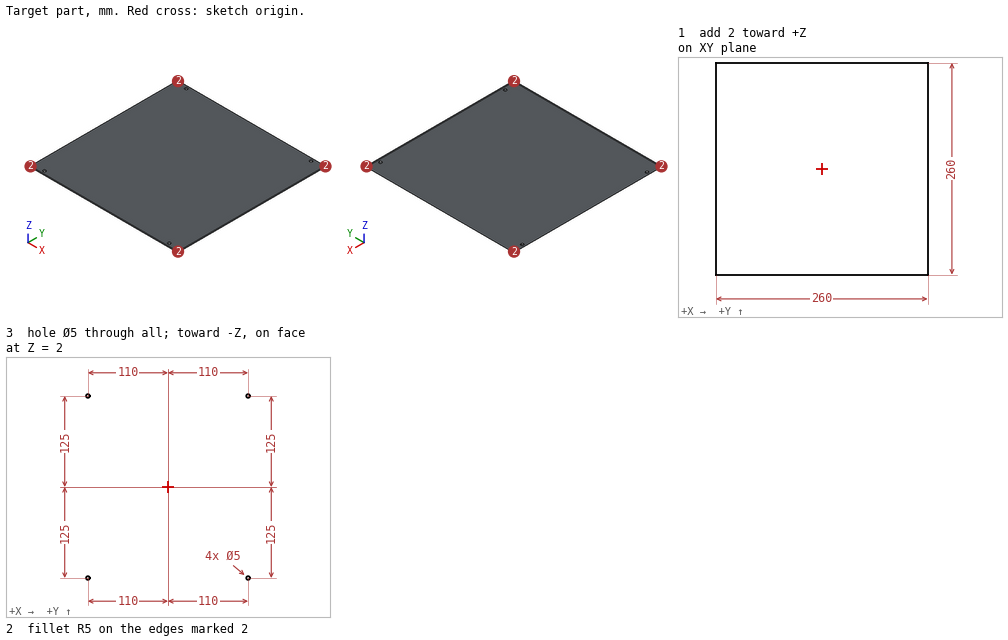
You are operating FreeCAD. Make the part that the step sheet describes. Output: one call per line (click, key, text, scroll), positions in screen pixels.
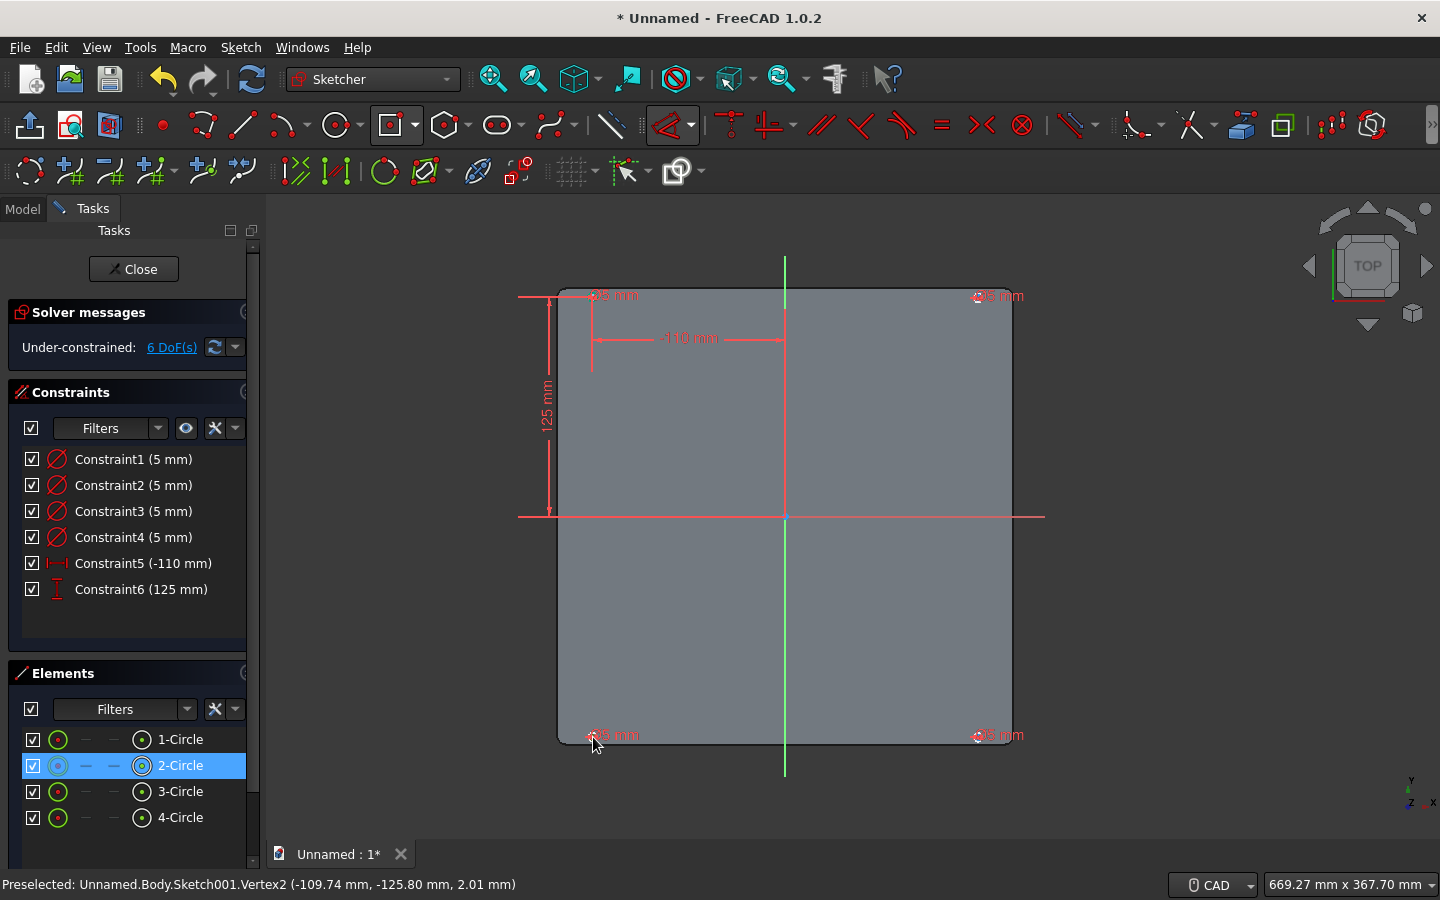
click(694, 126)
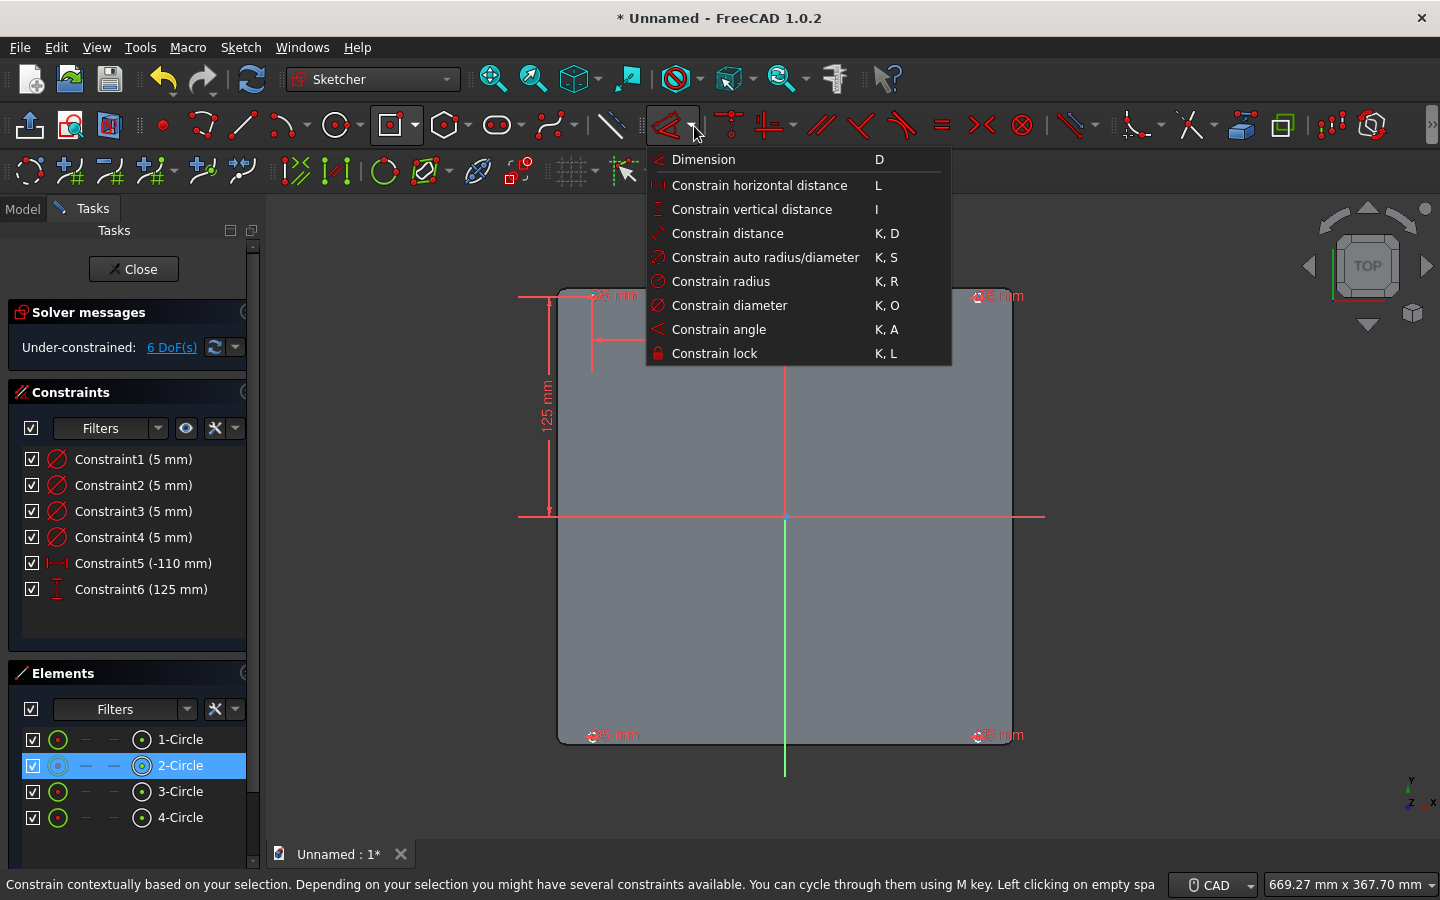
click(799, 185)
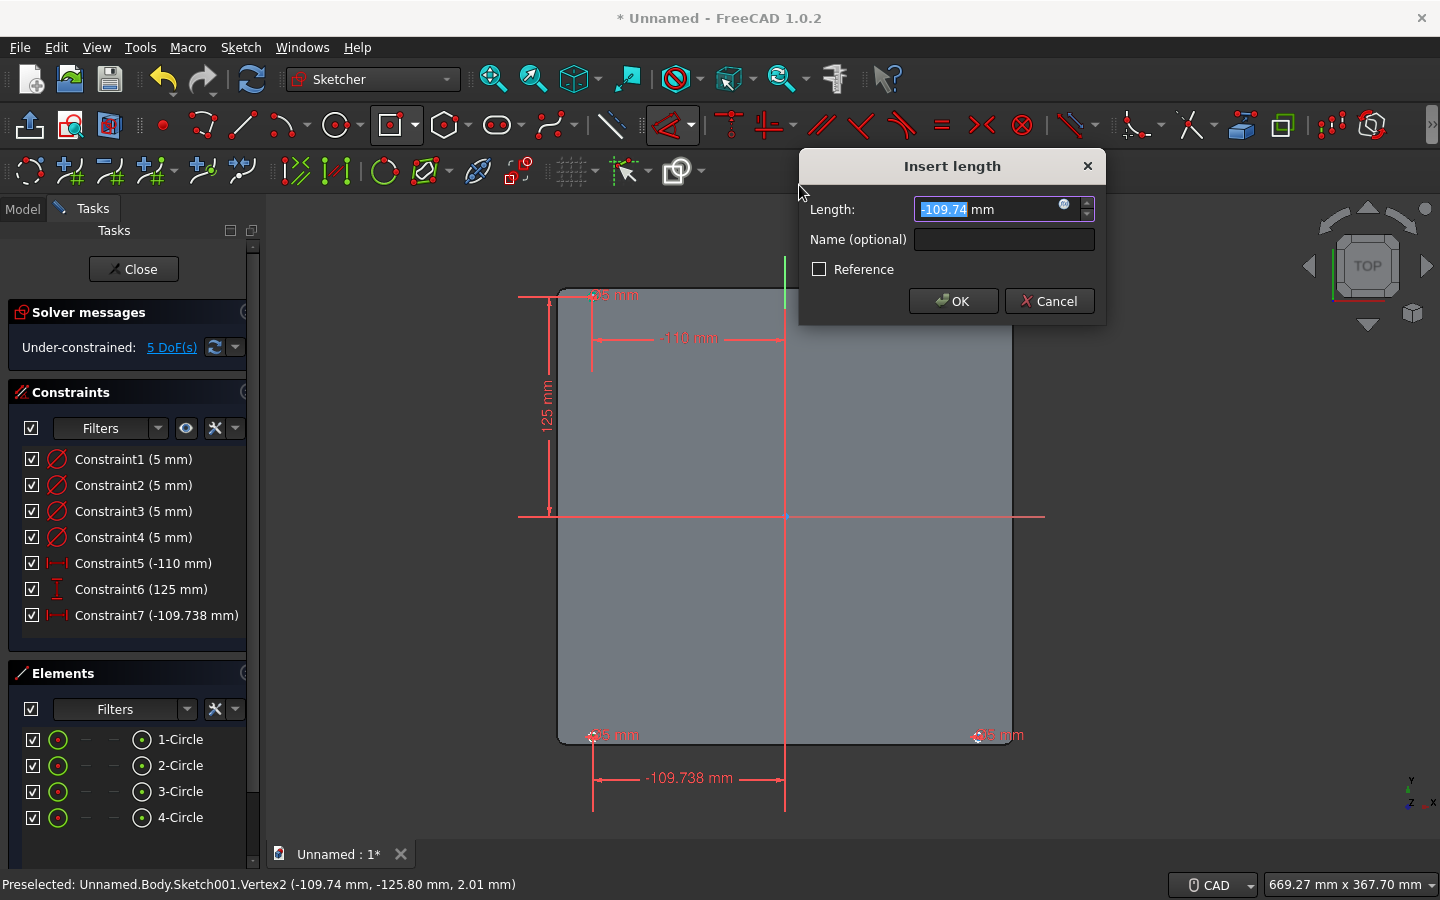
text(-110)
key(Return)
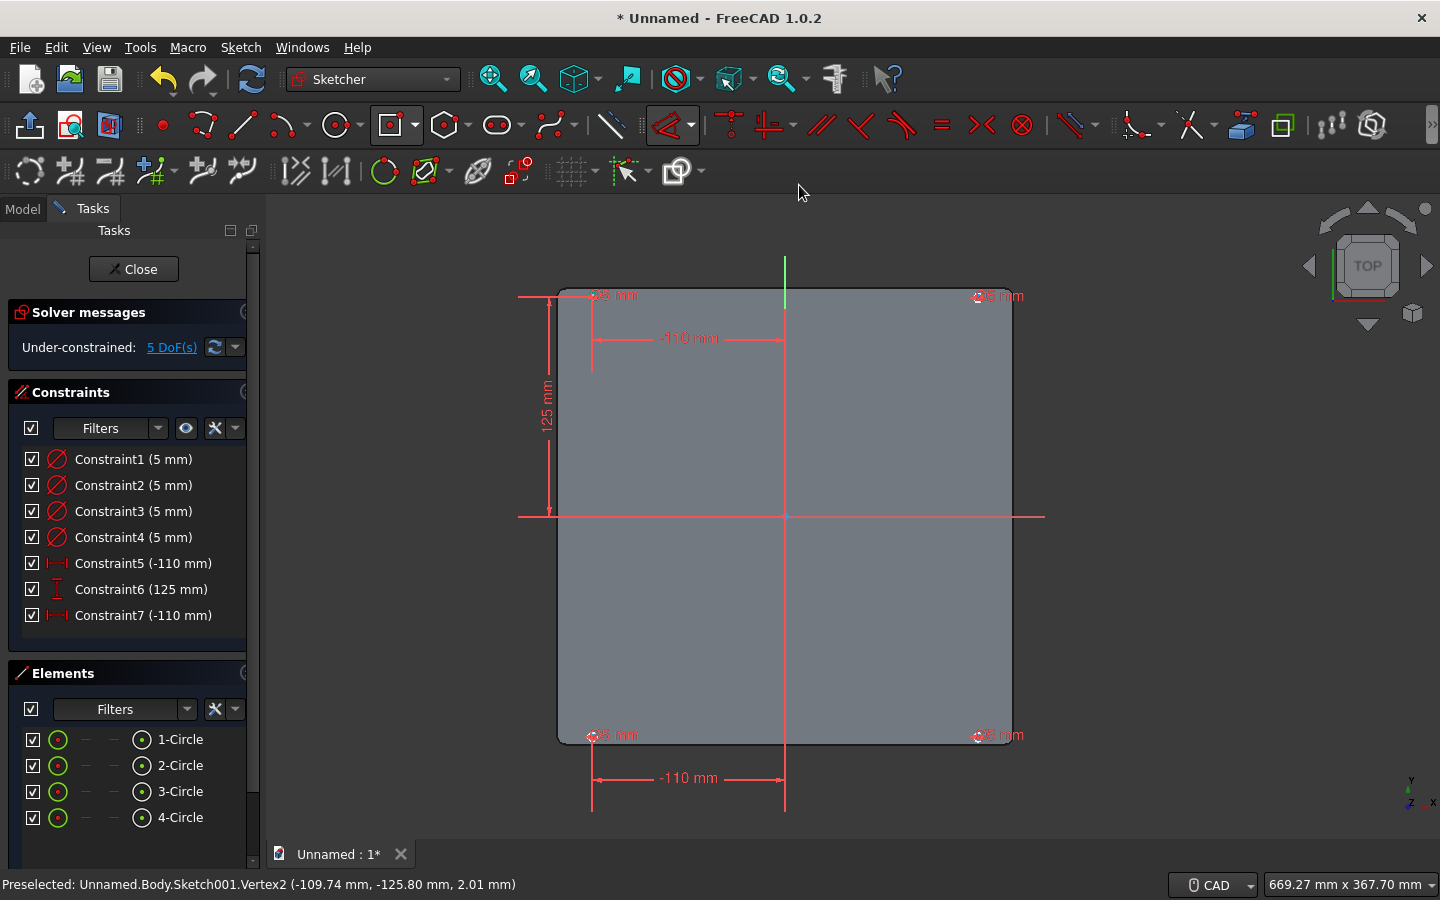
click(592, 737)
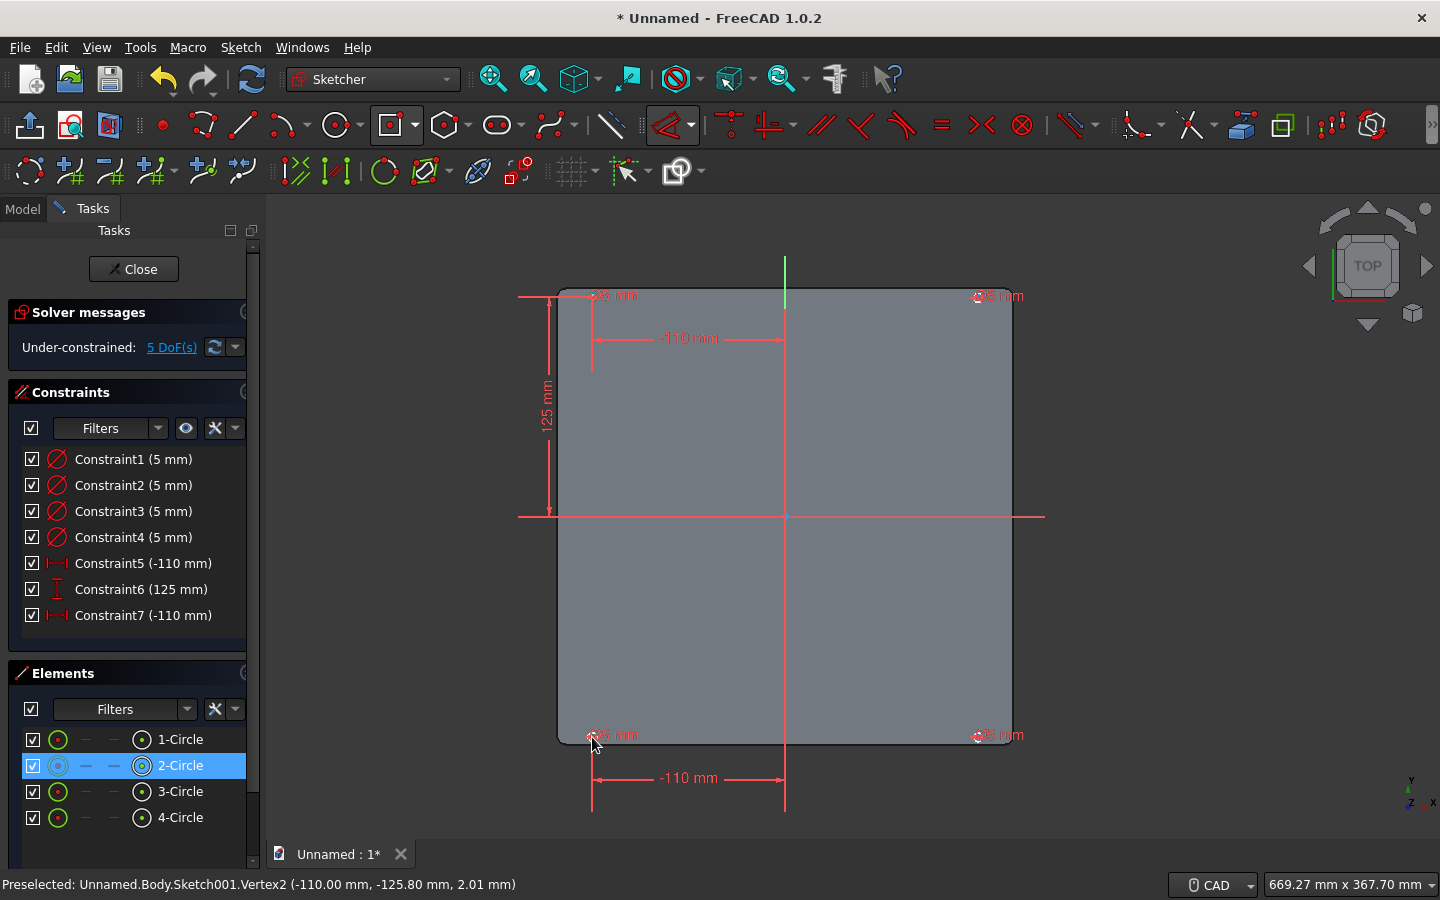
click(694, 126)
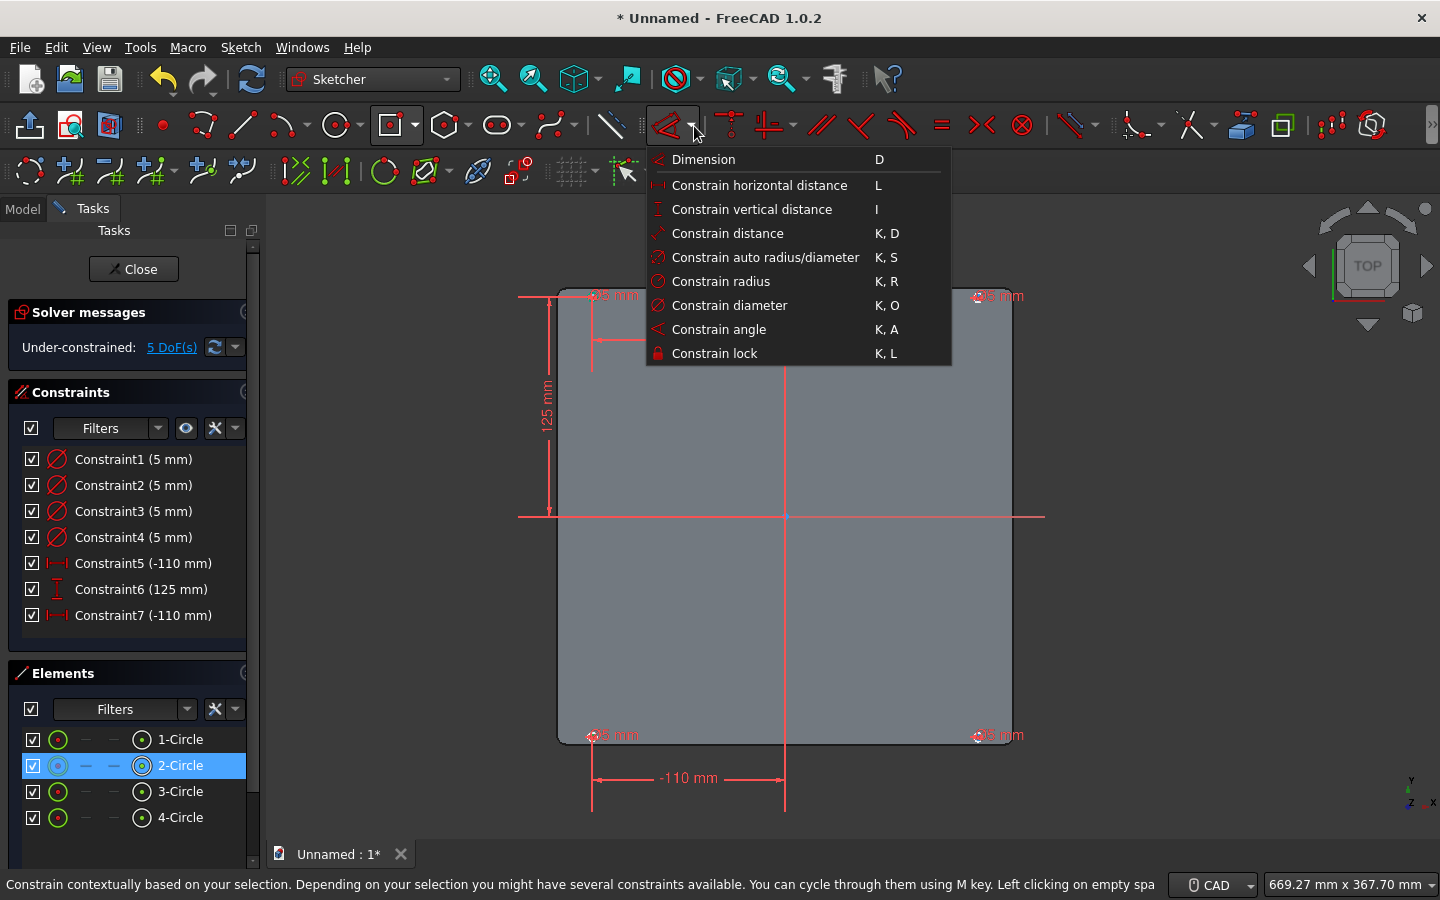
click(799, 209)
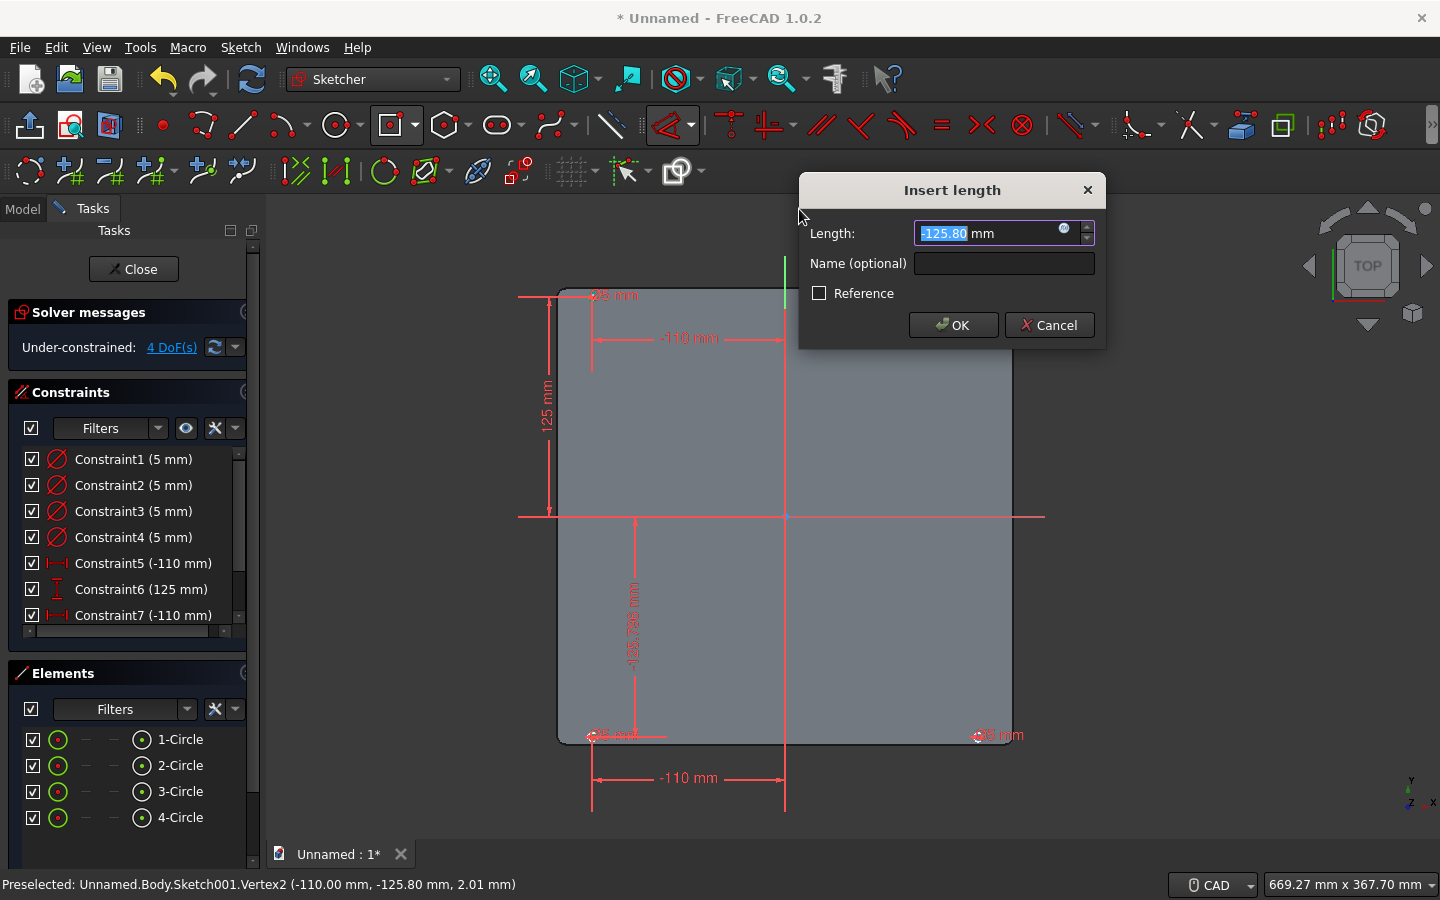
text(-125)
key(Return)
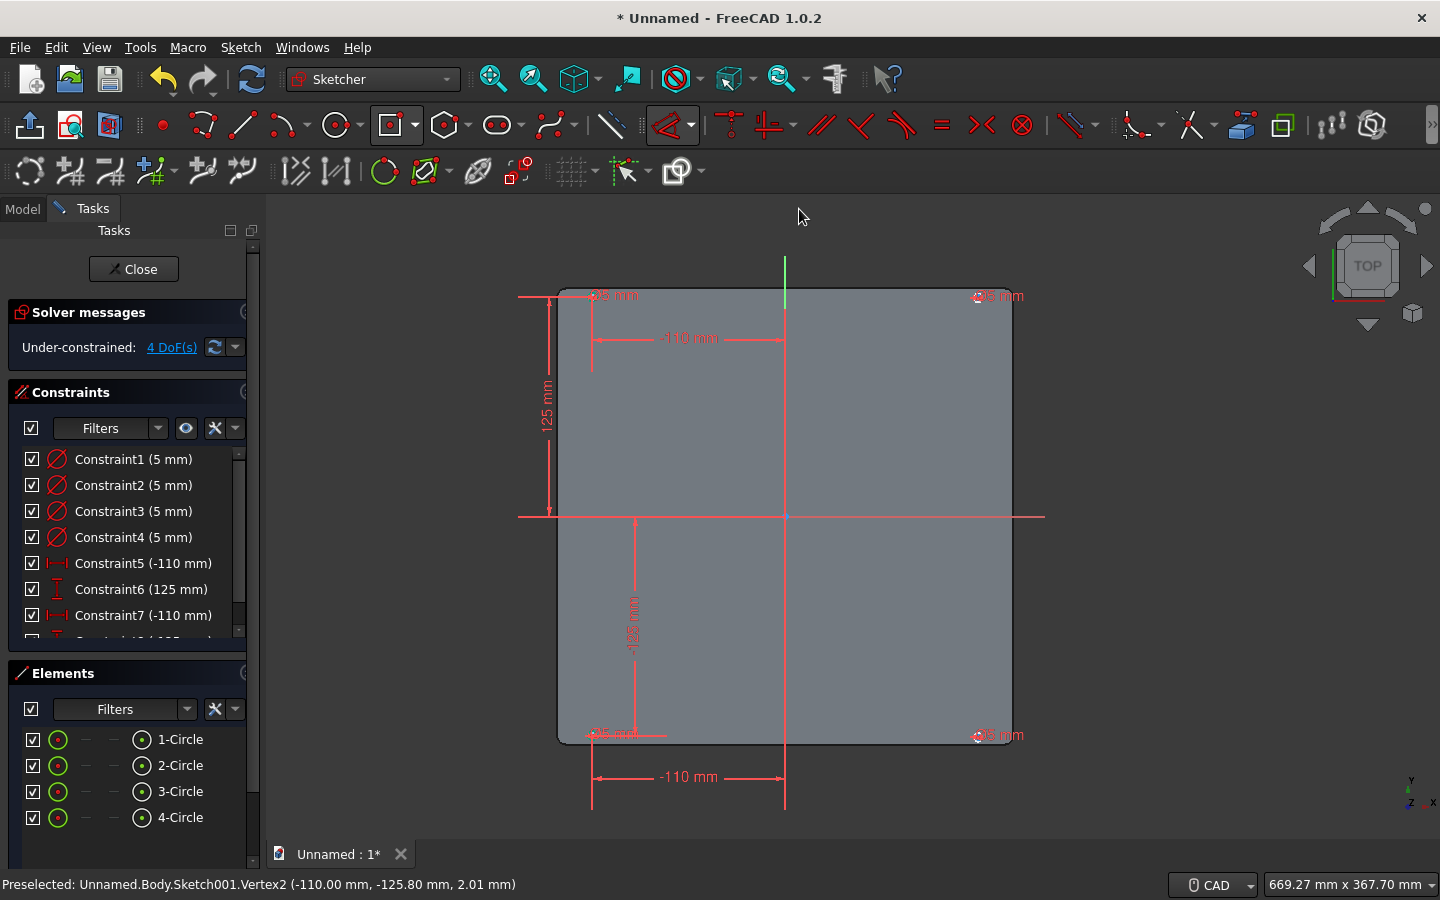
click(978, 737)